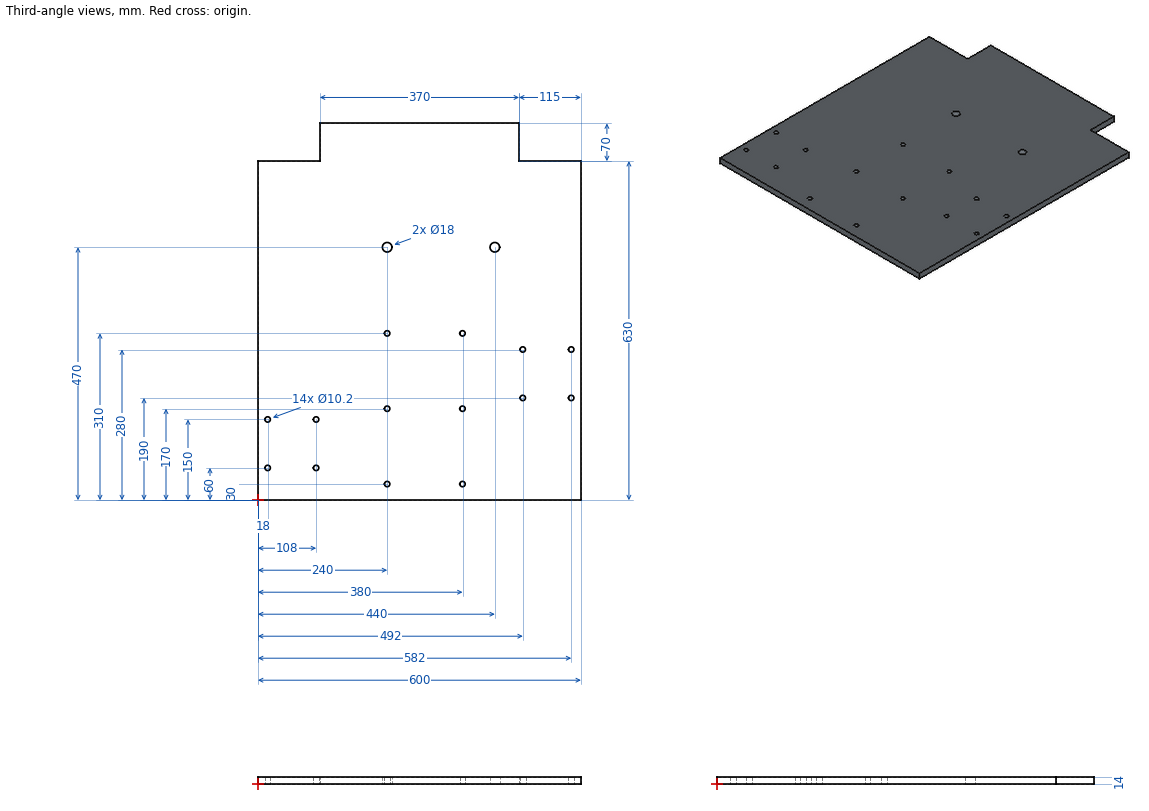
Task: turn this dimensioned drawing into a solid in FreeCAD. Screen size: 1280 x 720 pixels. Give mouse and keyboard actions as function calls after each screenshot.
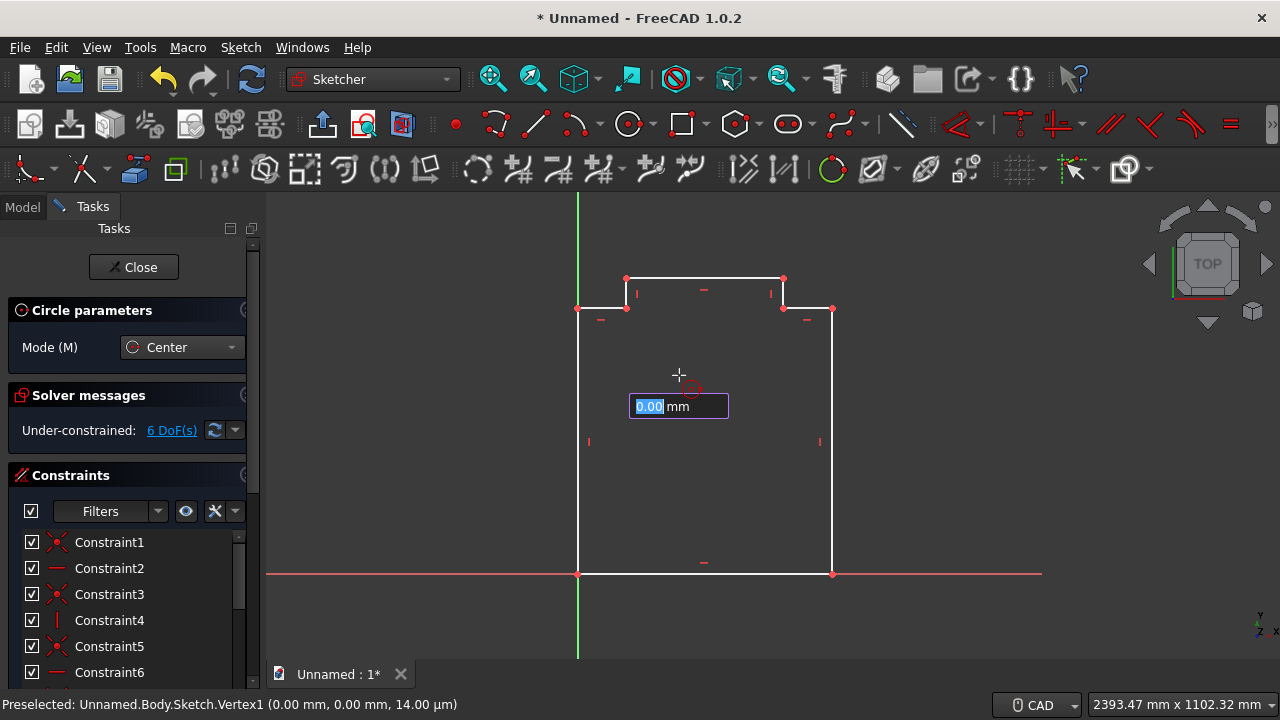
scroll(682, 372, up, 8)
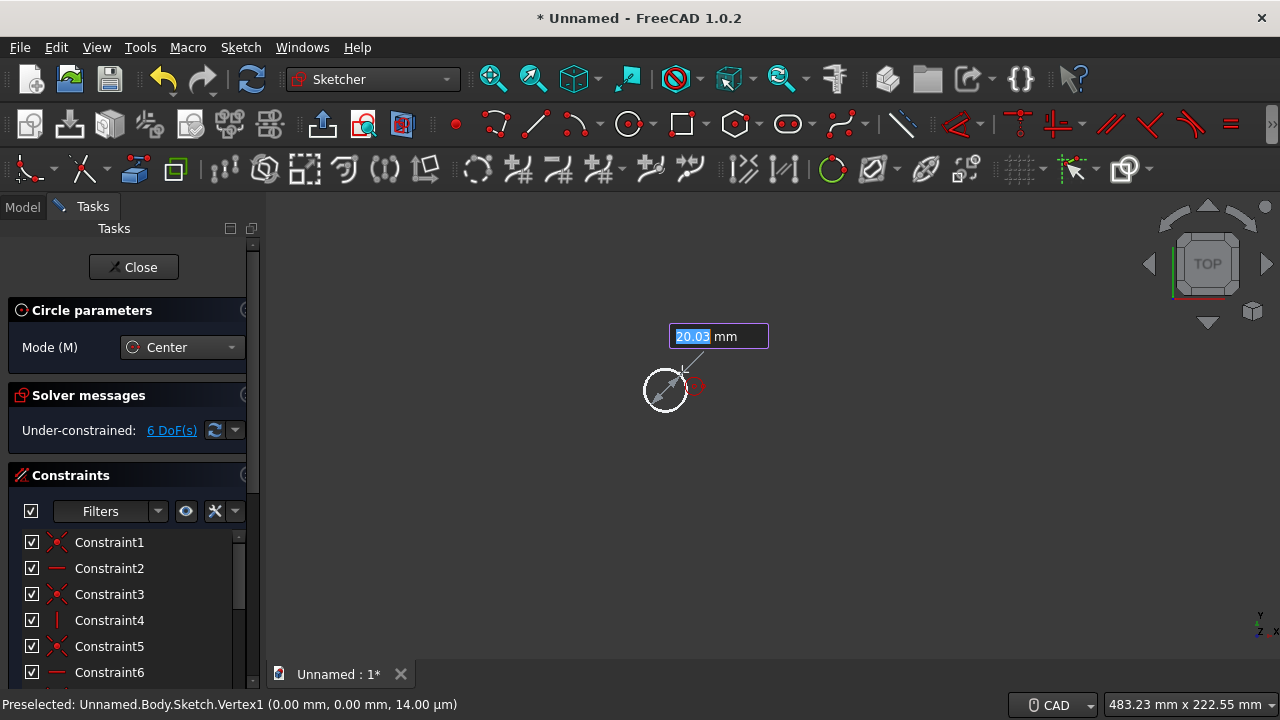
click(681, 372)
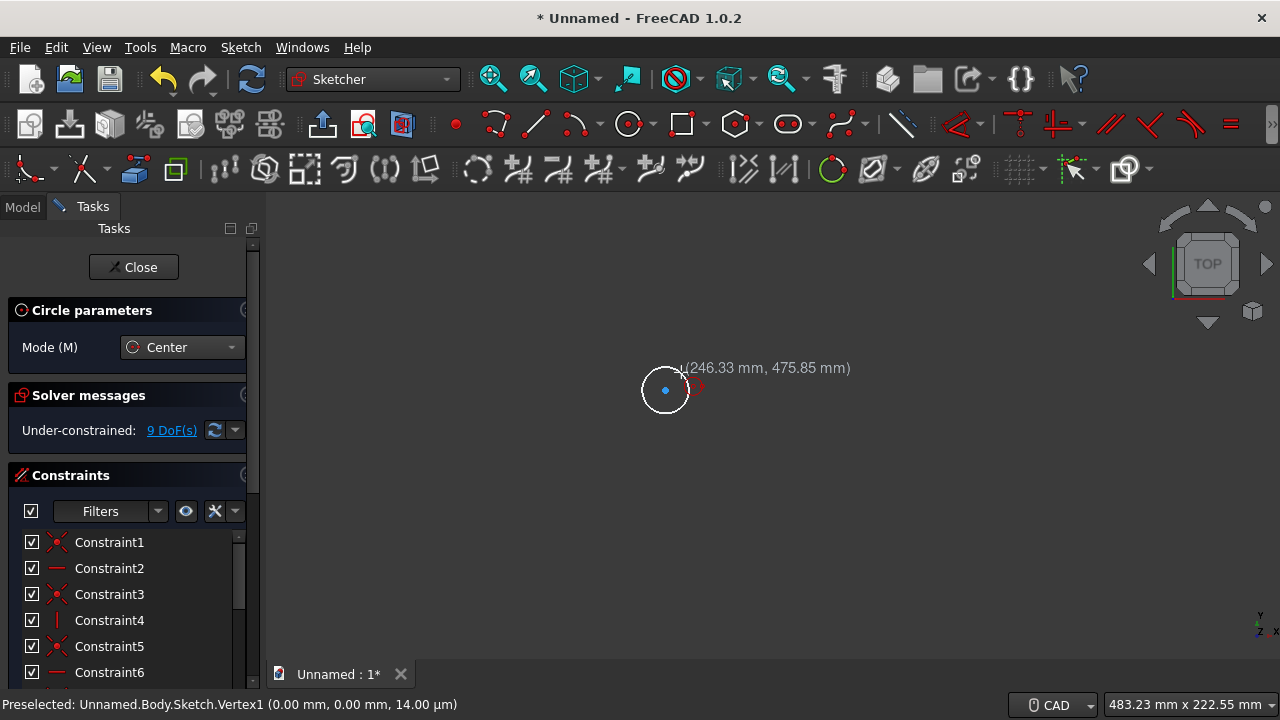
scroll(682, 372, down, 8)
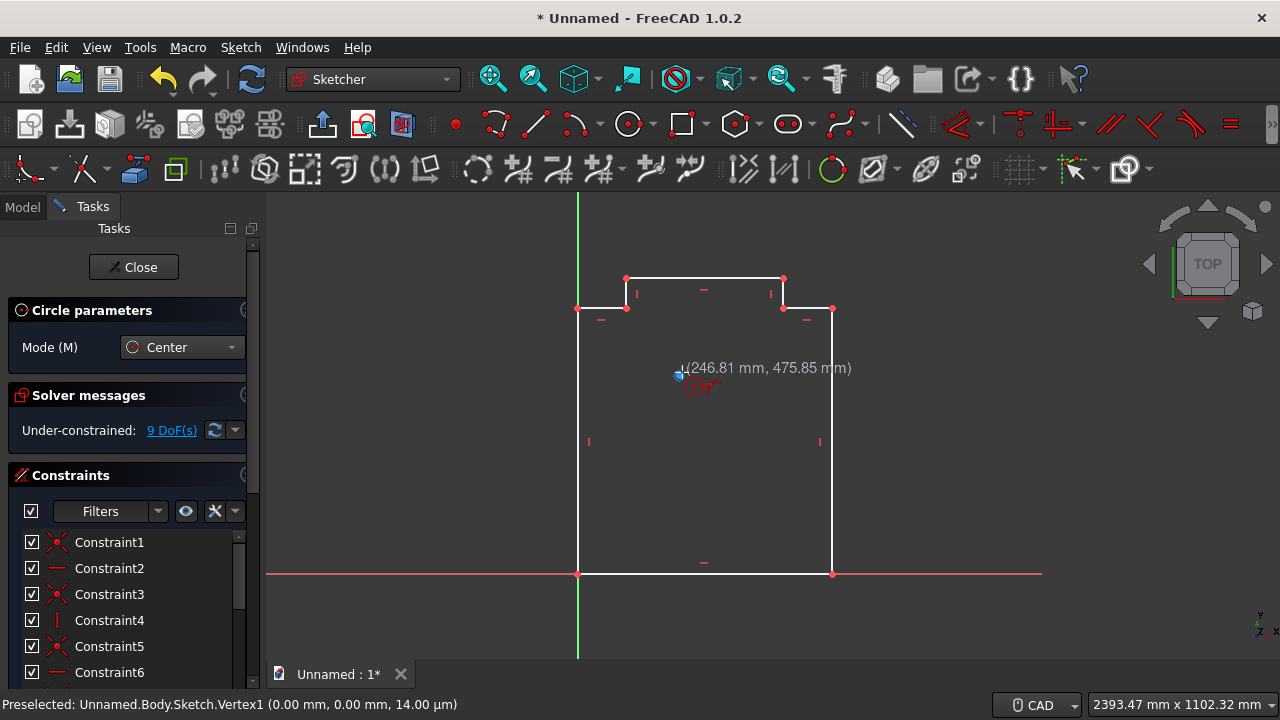
click(764, 375)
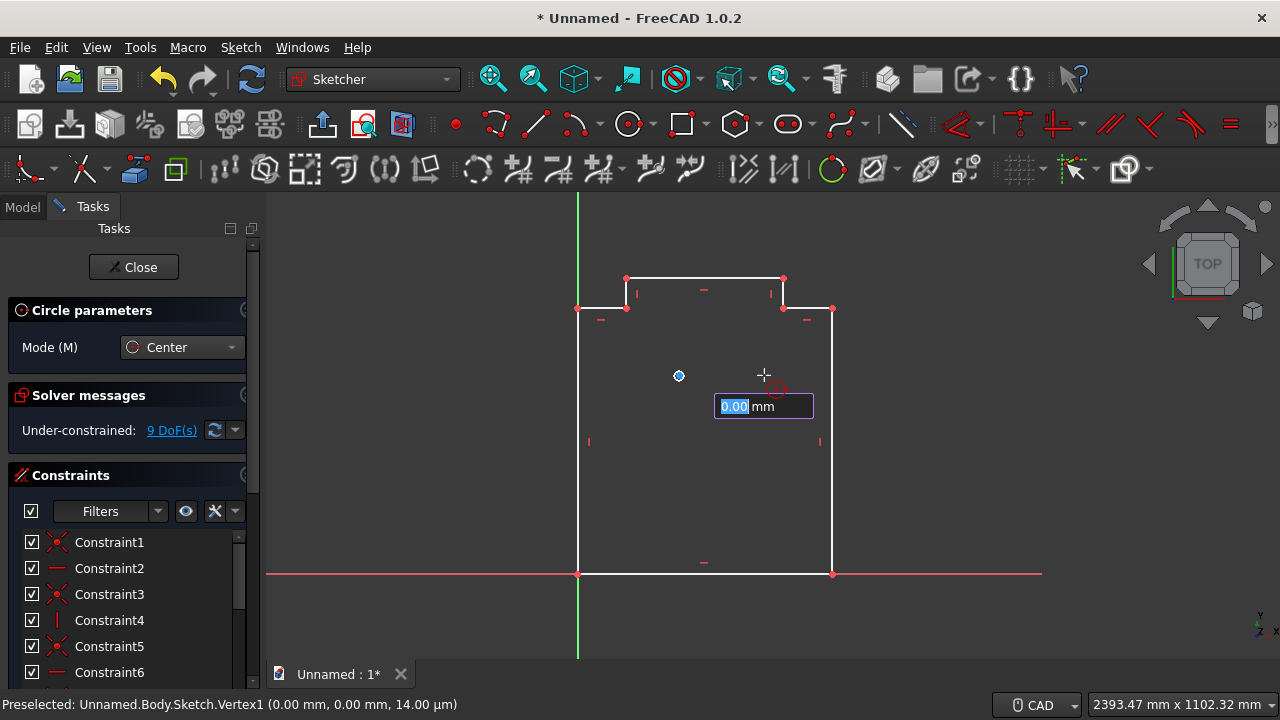
scroll(767, 372, up, 8)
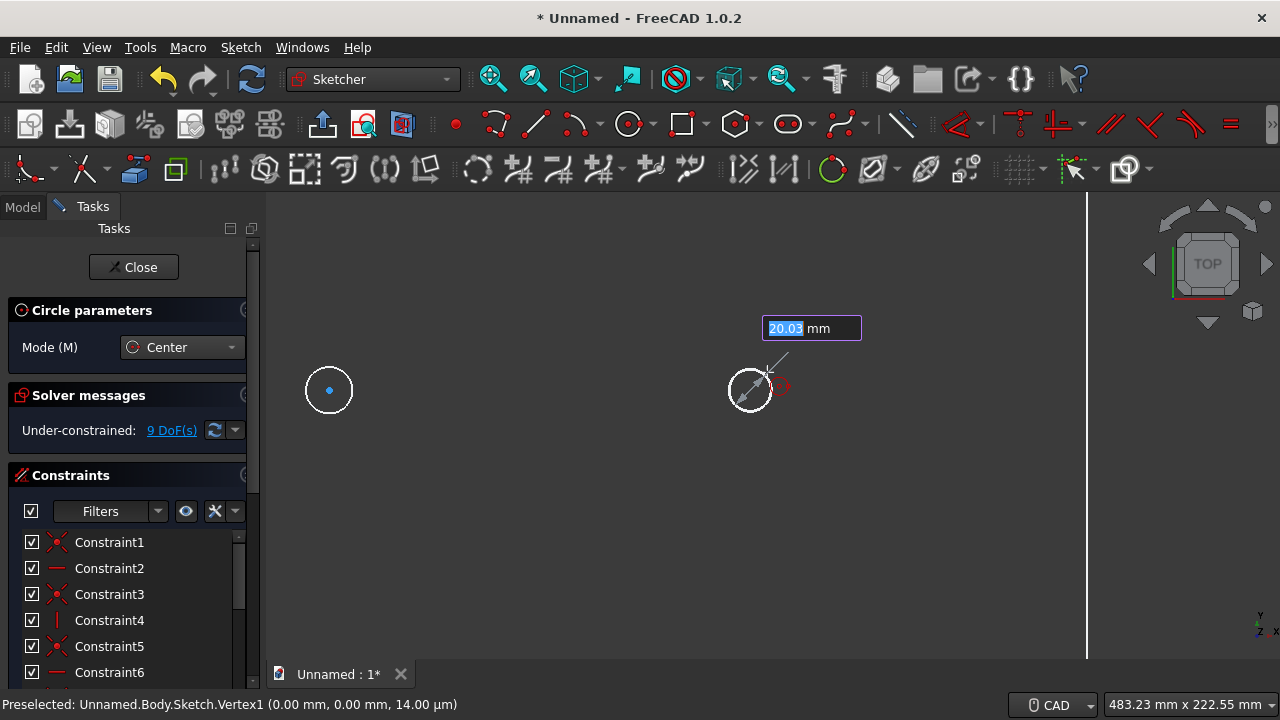
click(764, 372)
key(Escape)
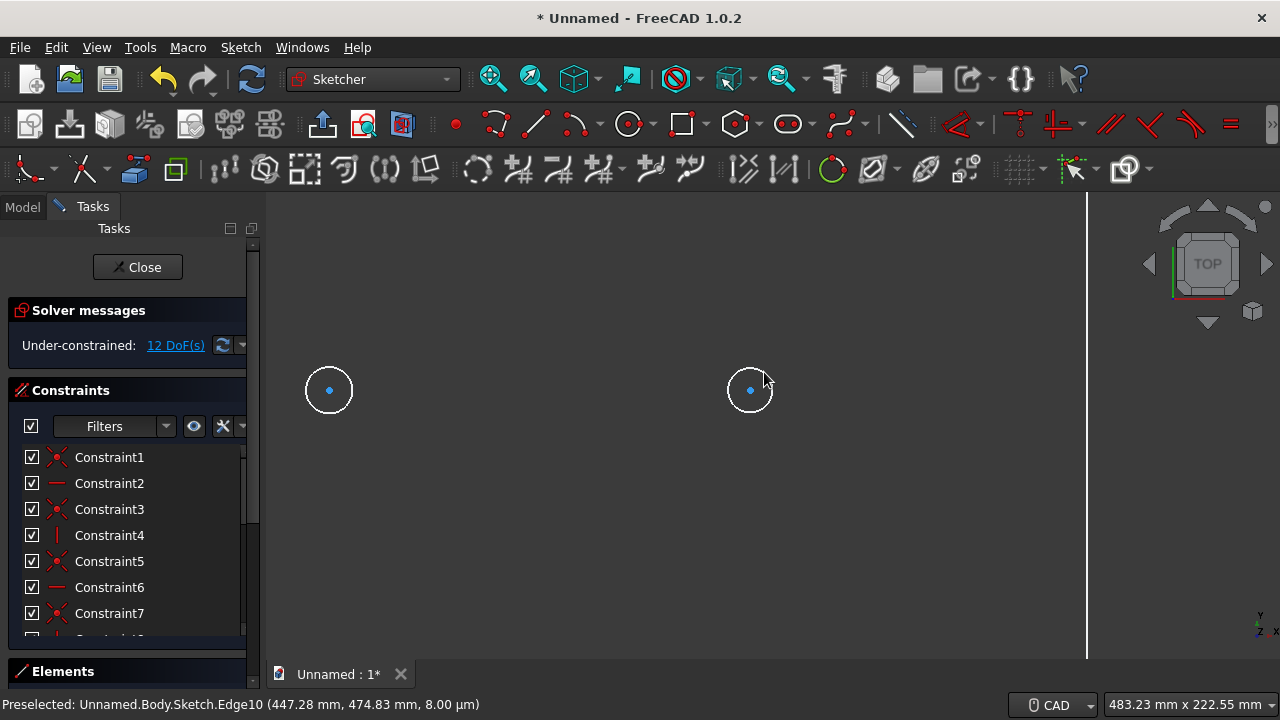
click(346, 374)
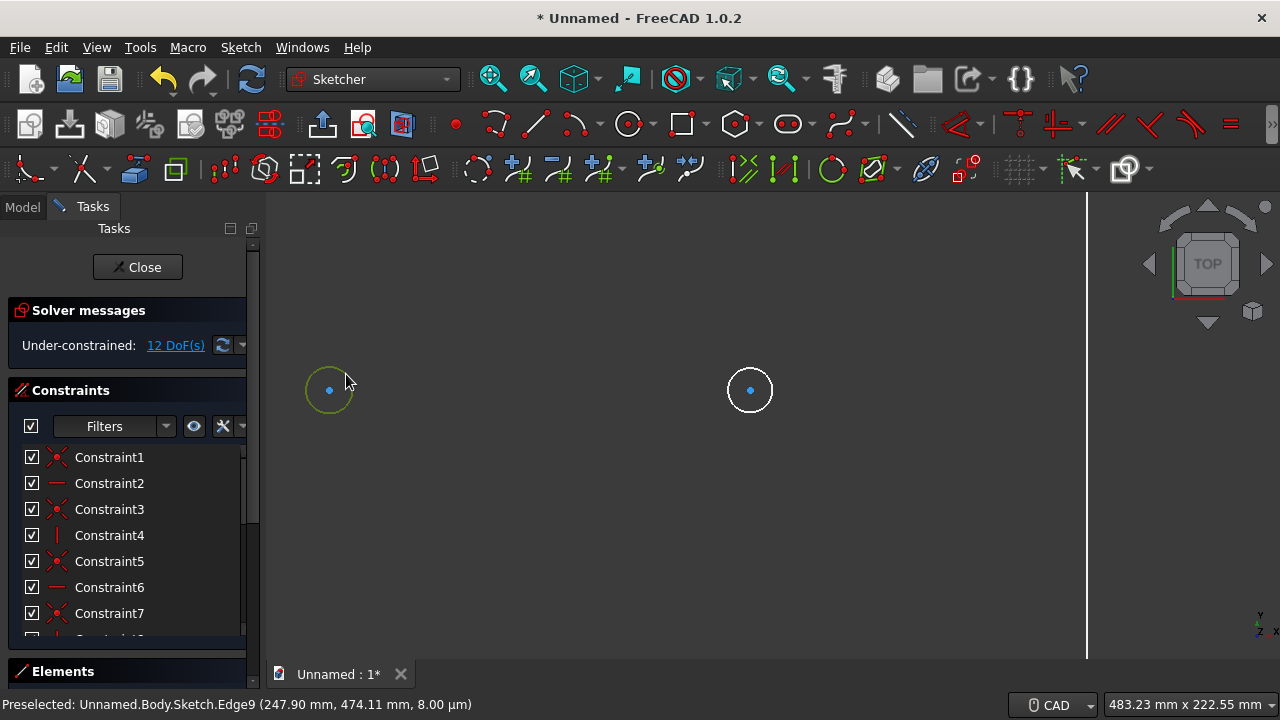
click(766, 375)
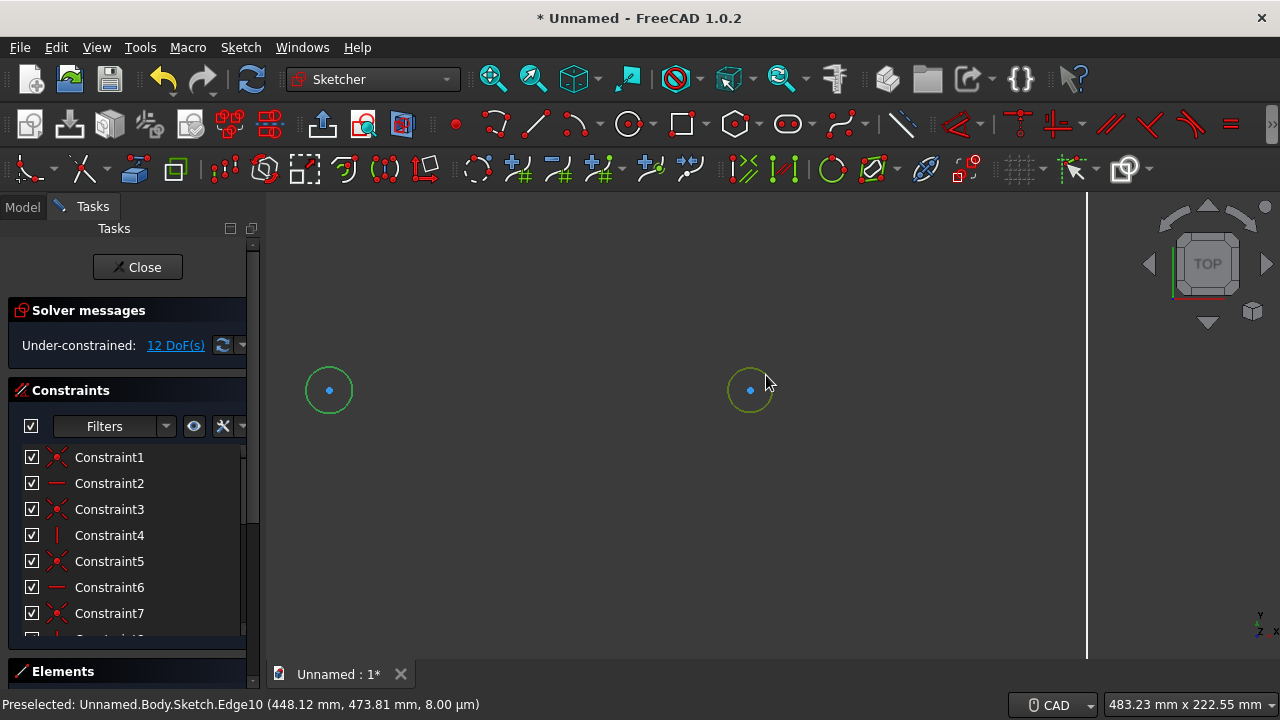
key(e)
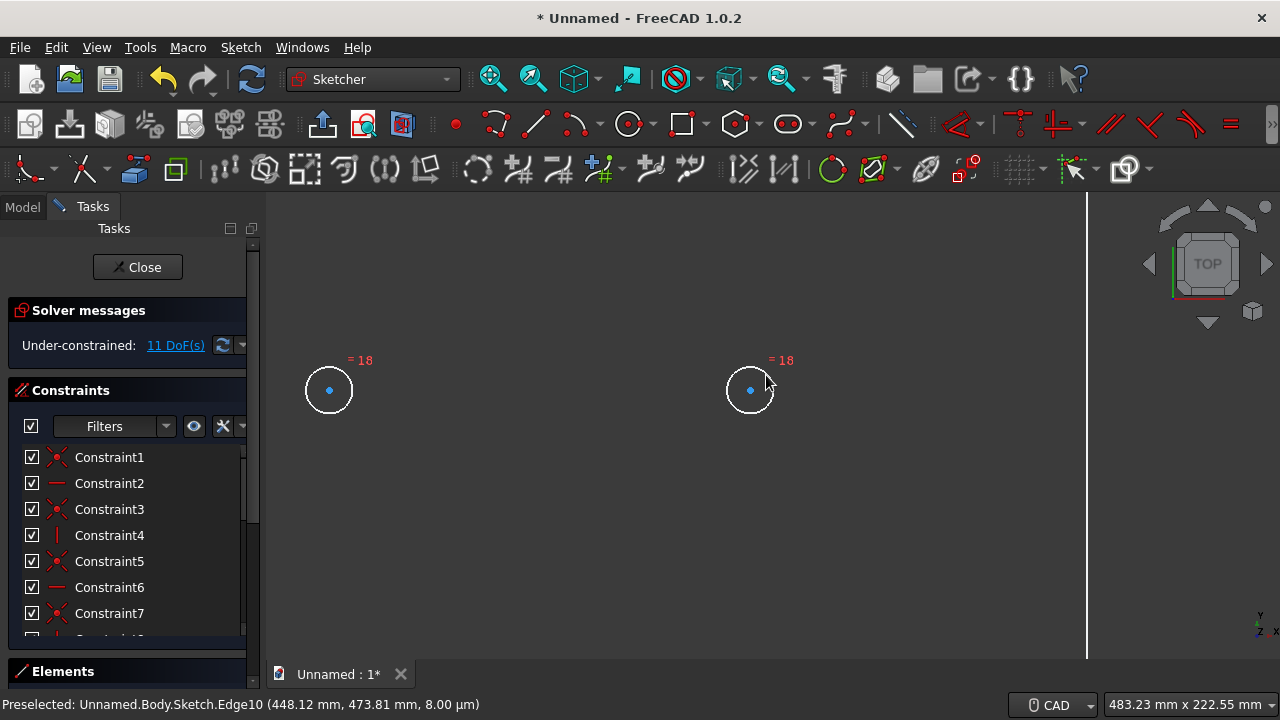
key(d)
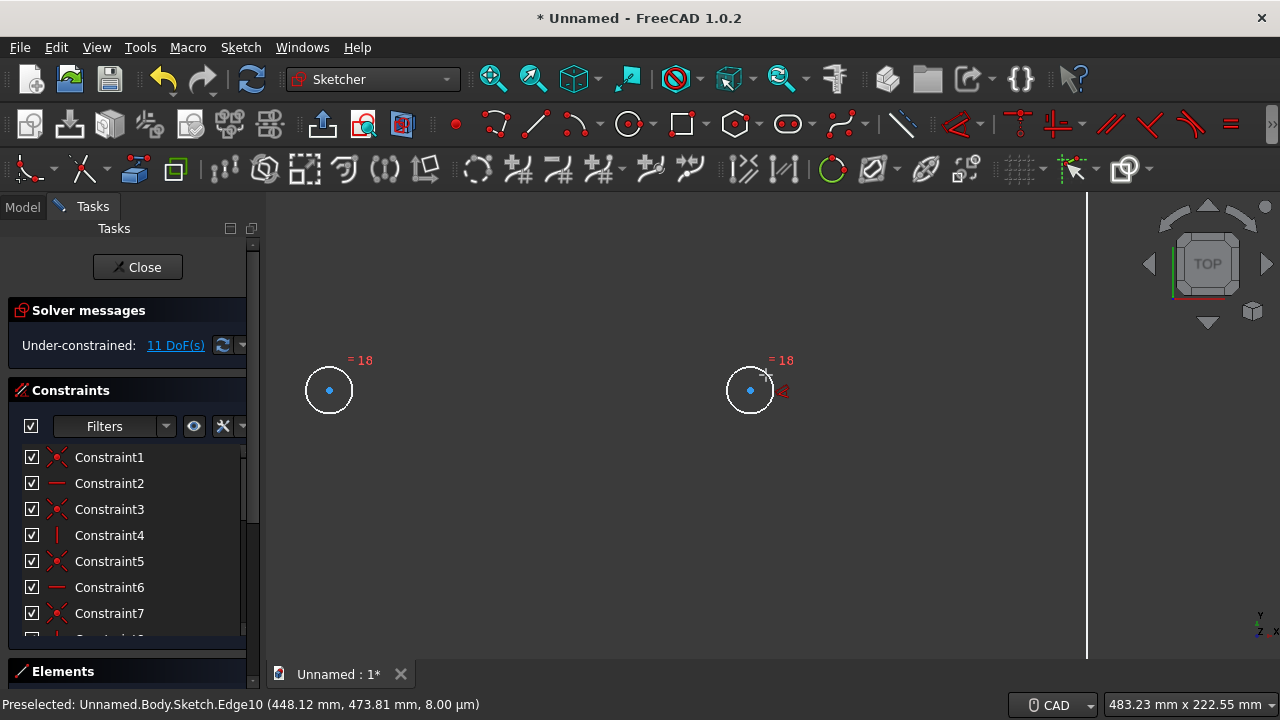
click(346, 374)
click(369, 352)